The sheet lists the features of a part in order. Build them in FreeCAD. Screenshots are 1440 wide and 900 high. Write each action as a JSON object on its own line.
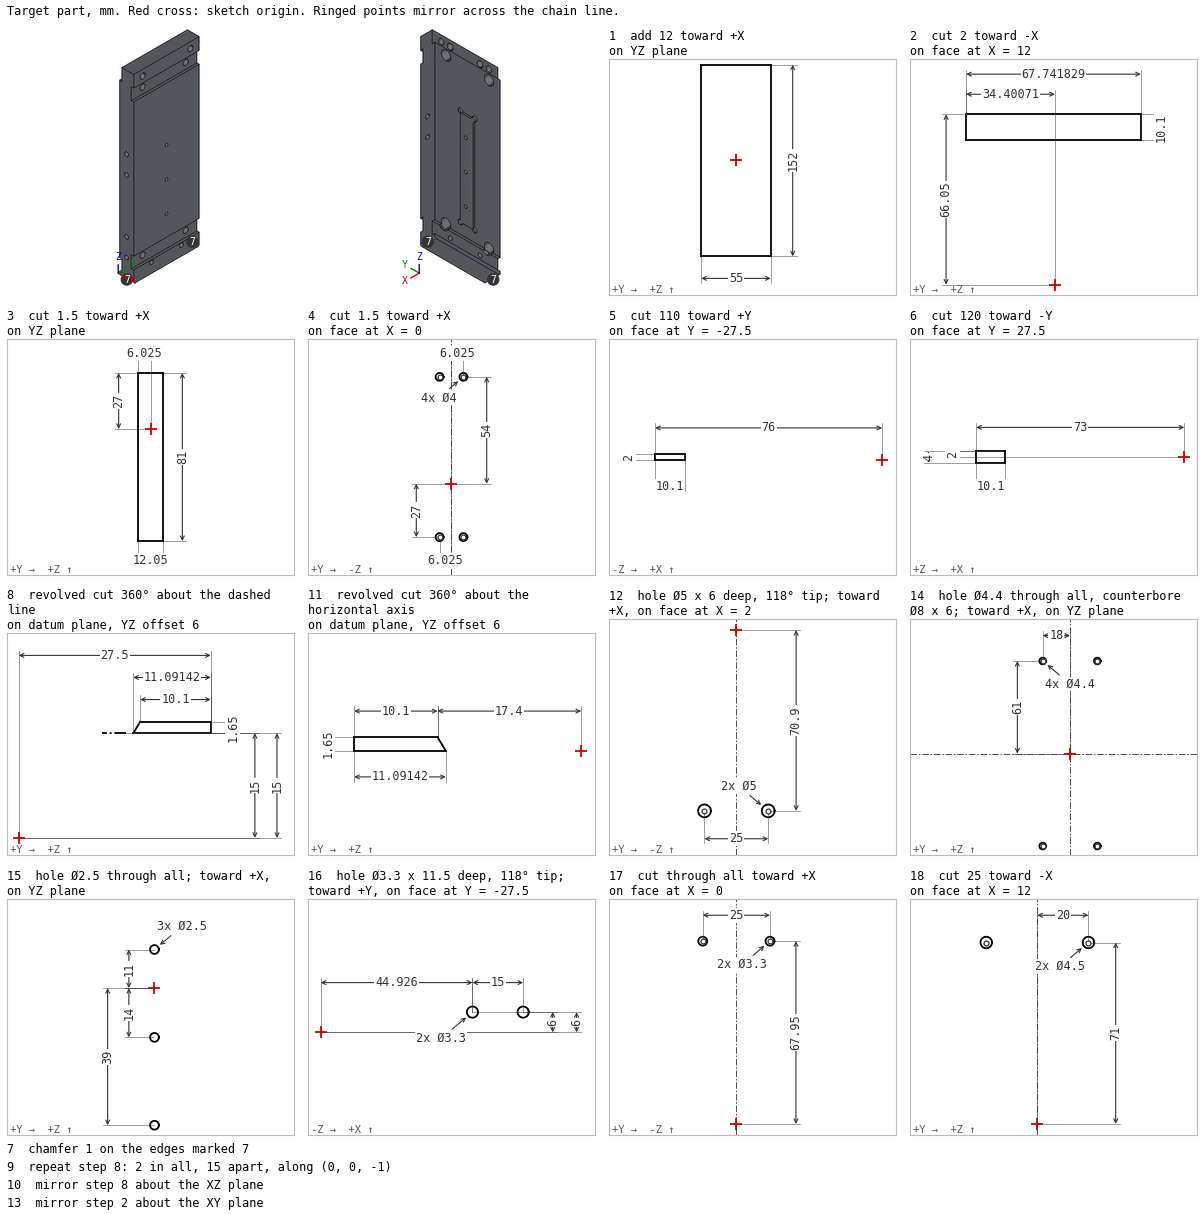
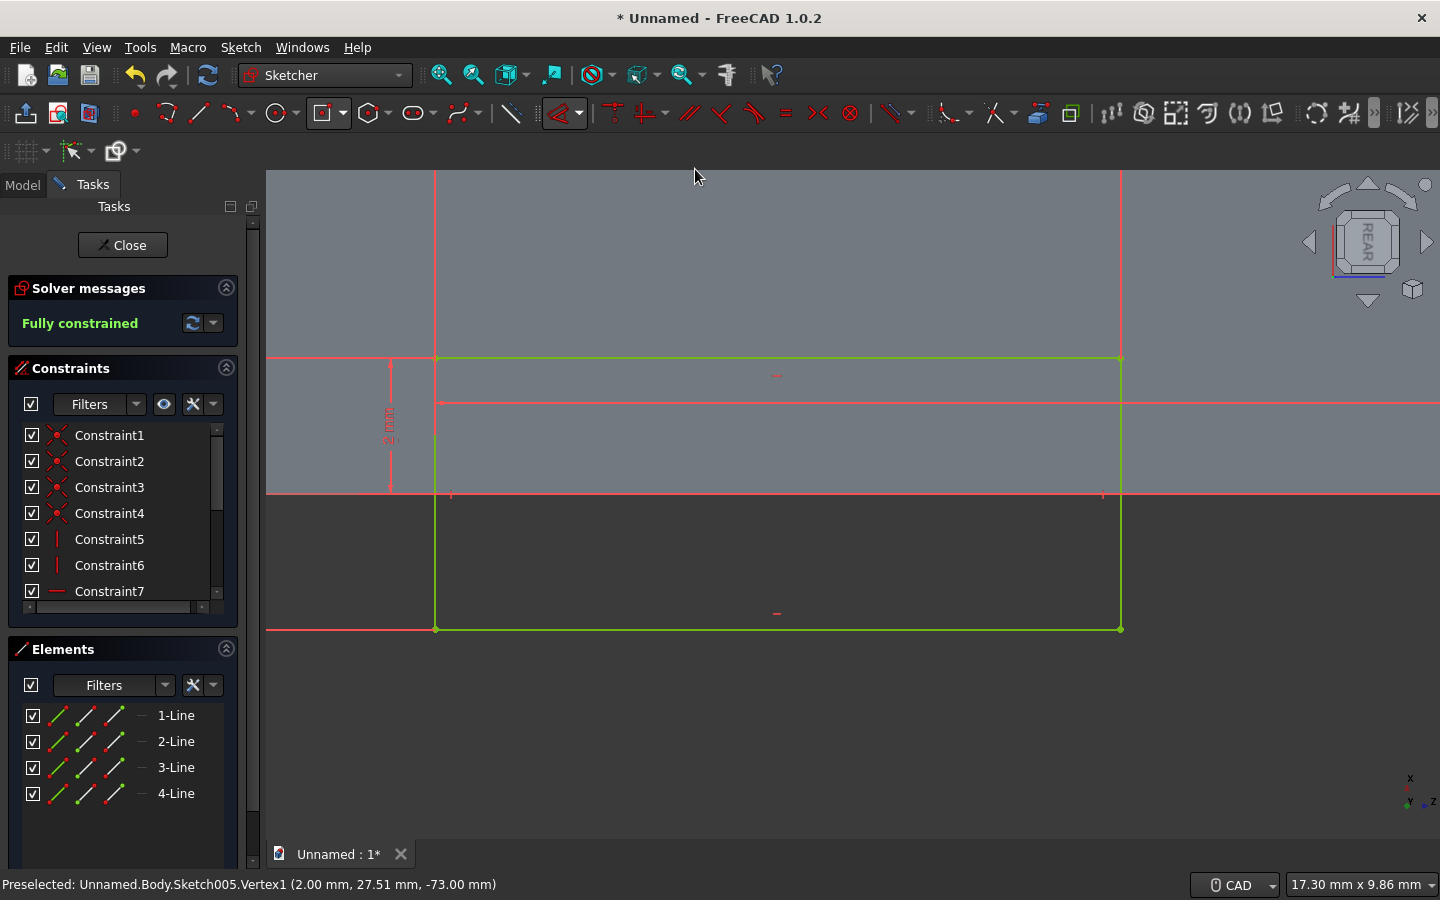
{"action": "left_click", "coordinate": [123, 245]}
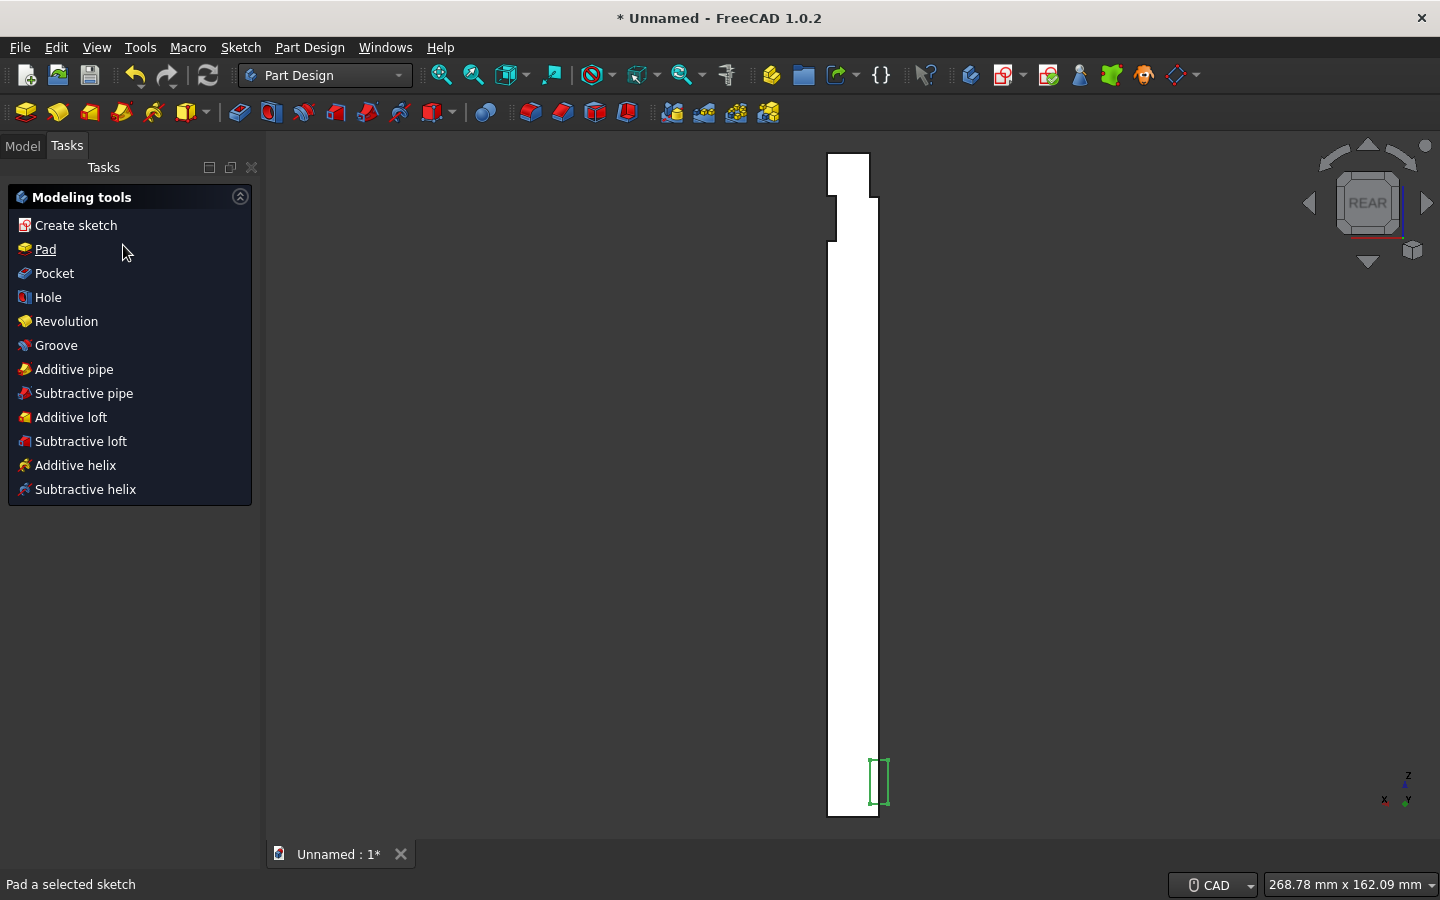
{"action": "left_click", "coordinate": [240, 112]}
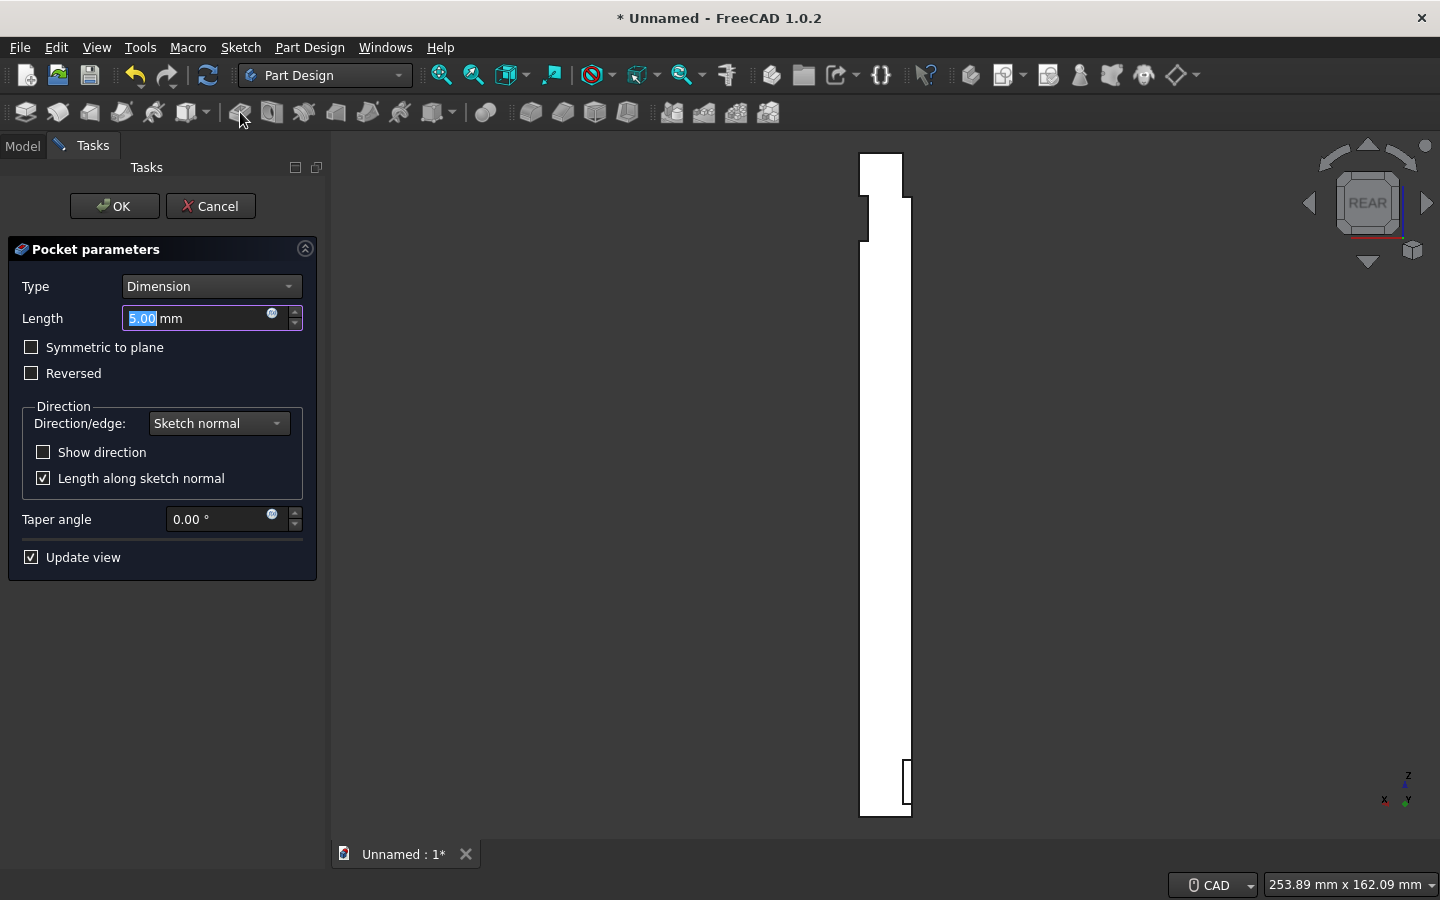
{"action": "type", "text": "120"}
{"action": "key", "text": "Tab"}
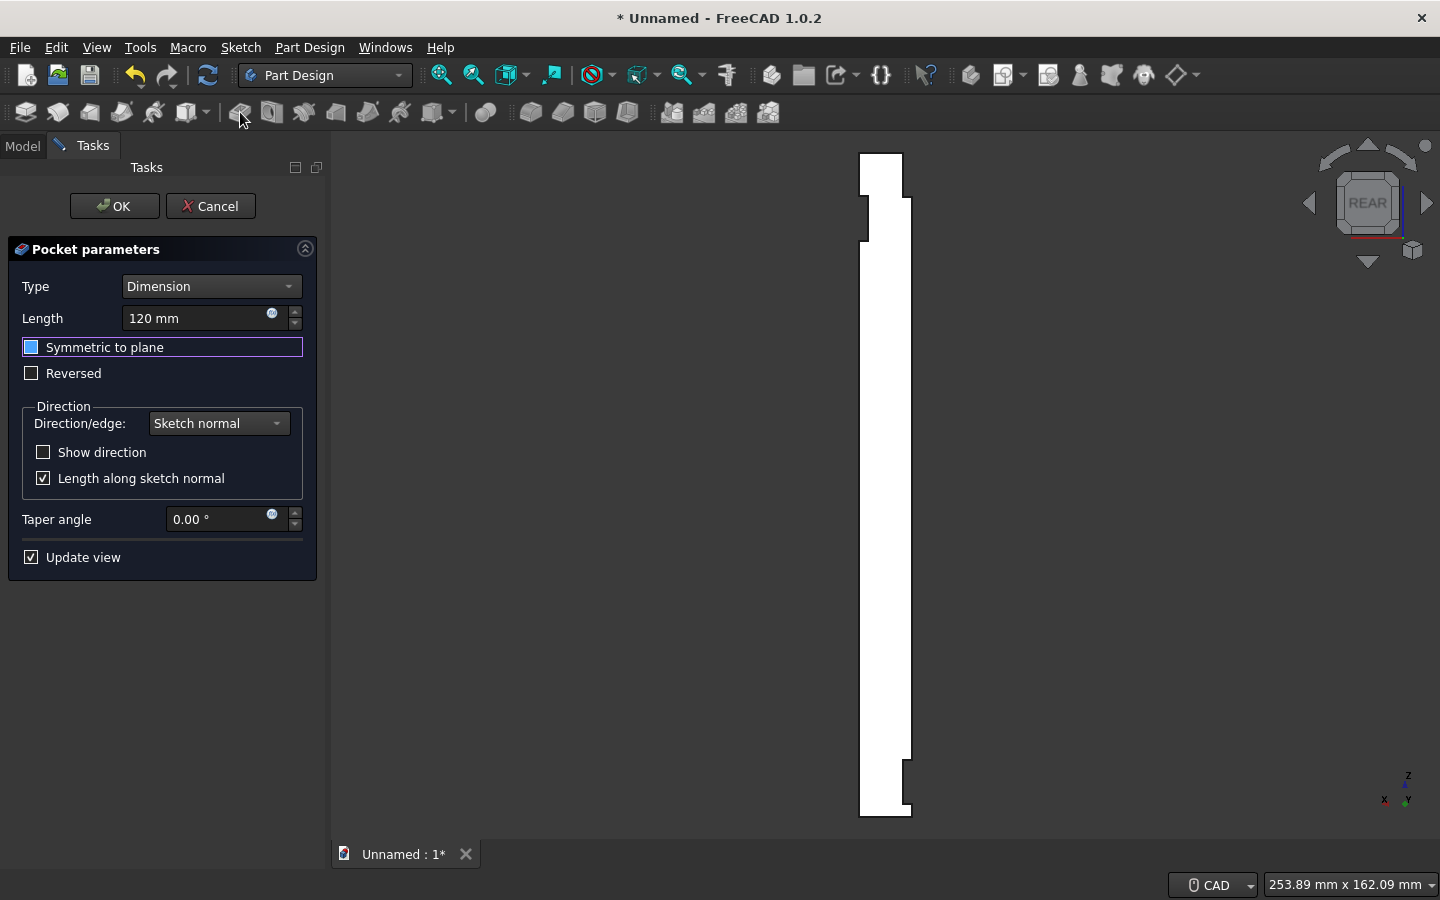
{"action": "left_click", "coordinate": [115, 206]}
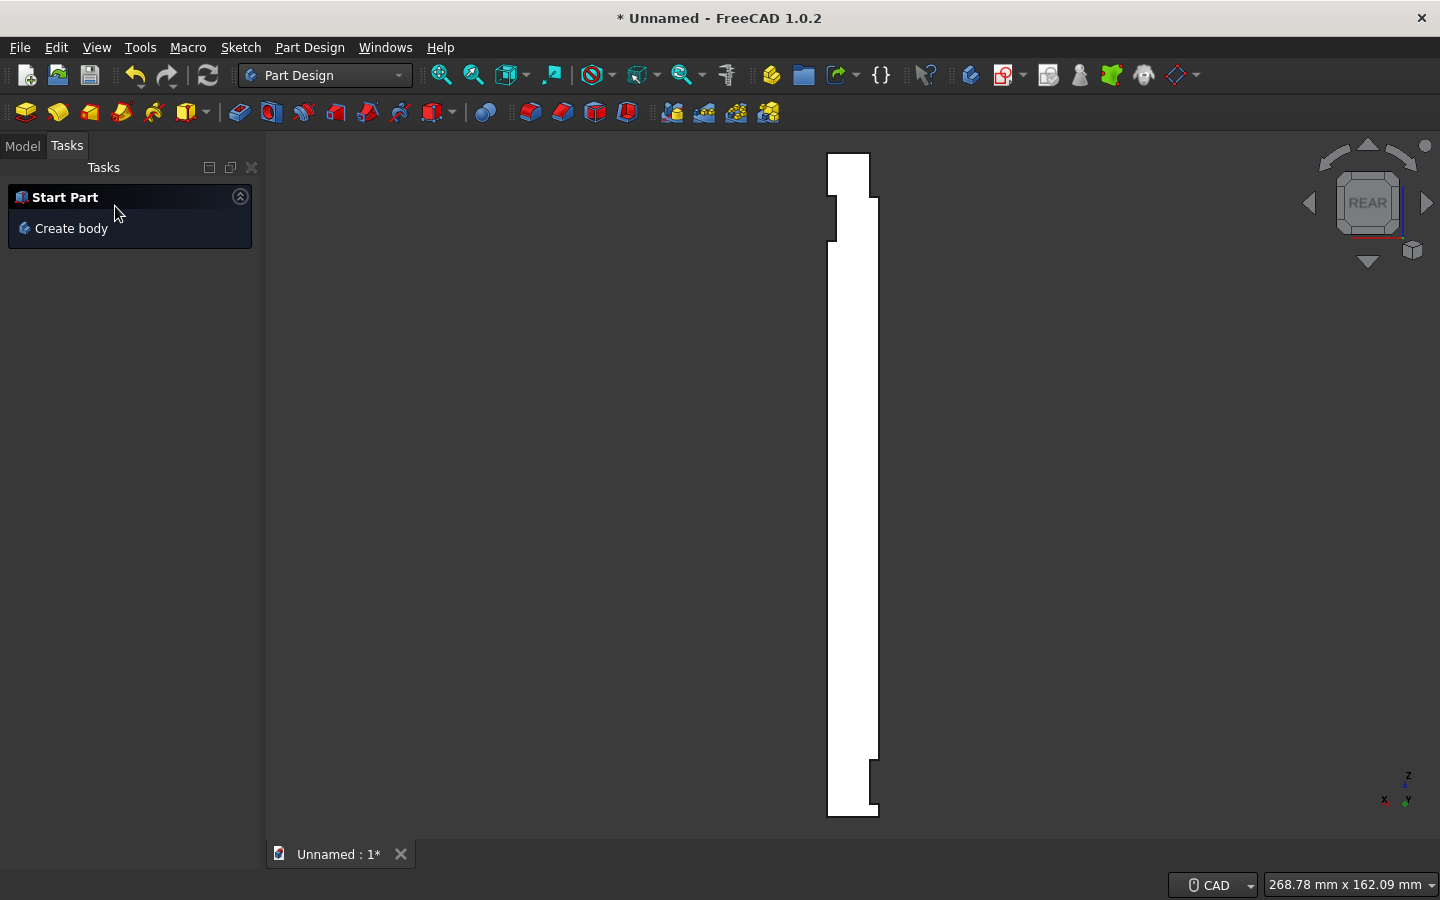
{"action": "key", "text": "0"}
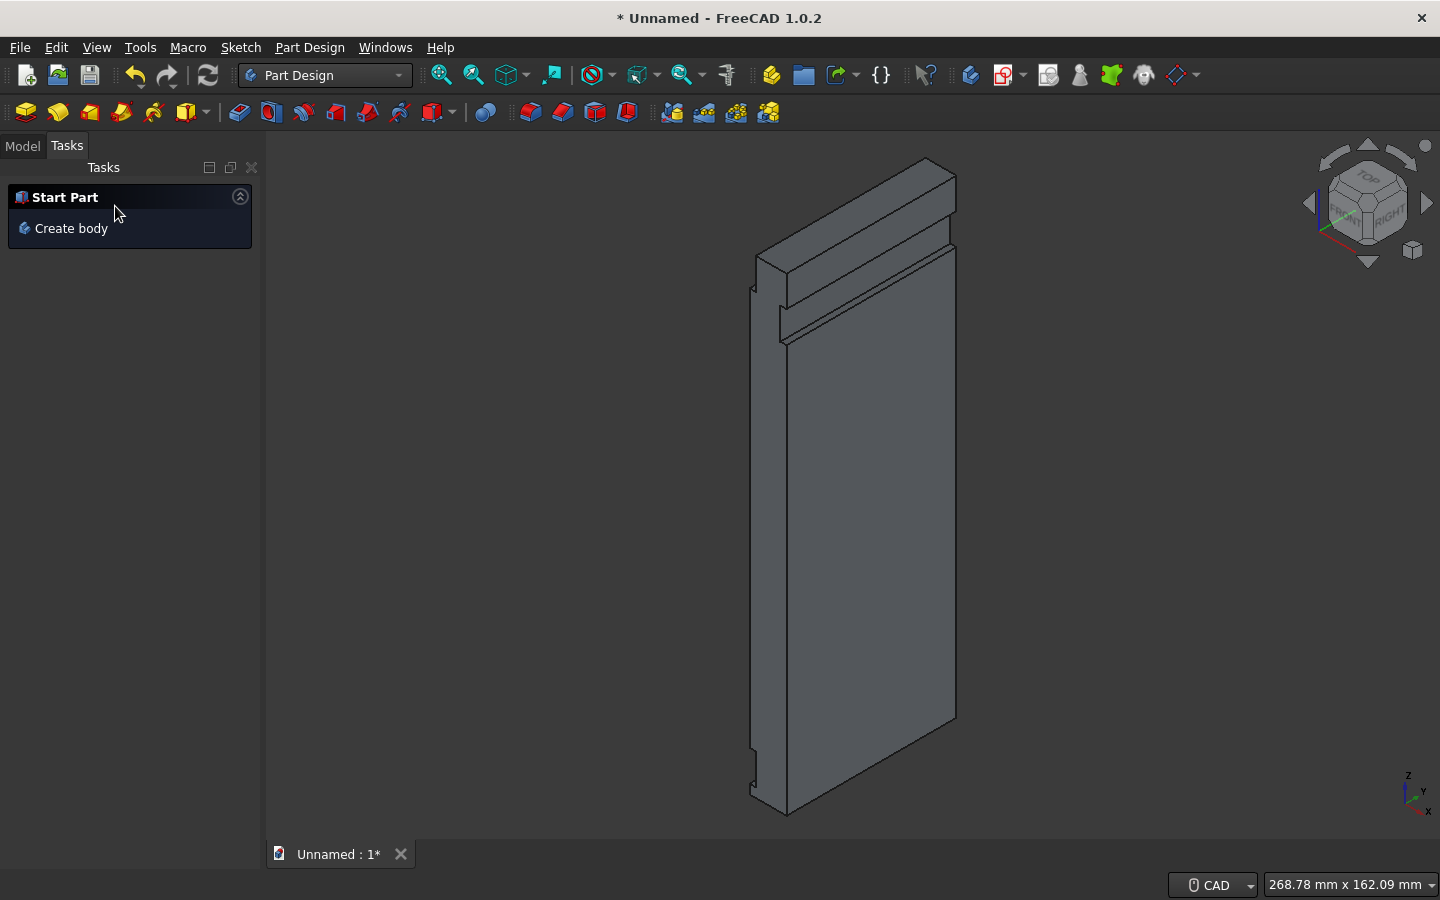
{"action": "key", "text": "2"}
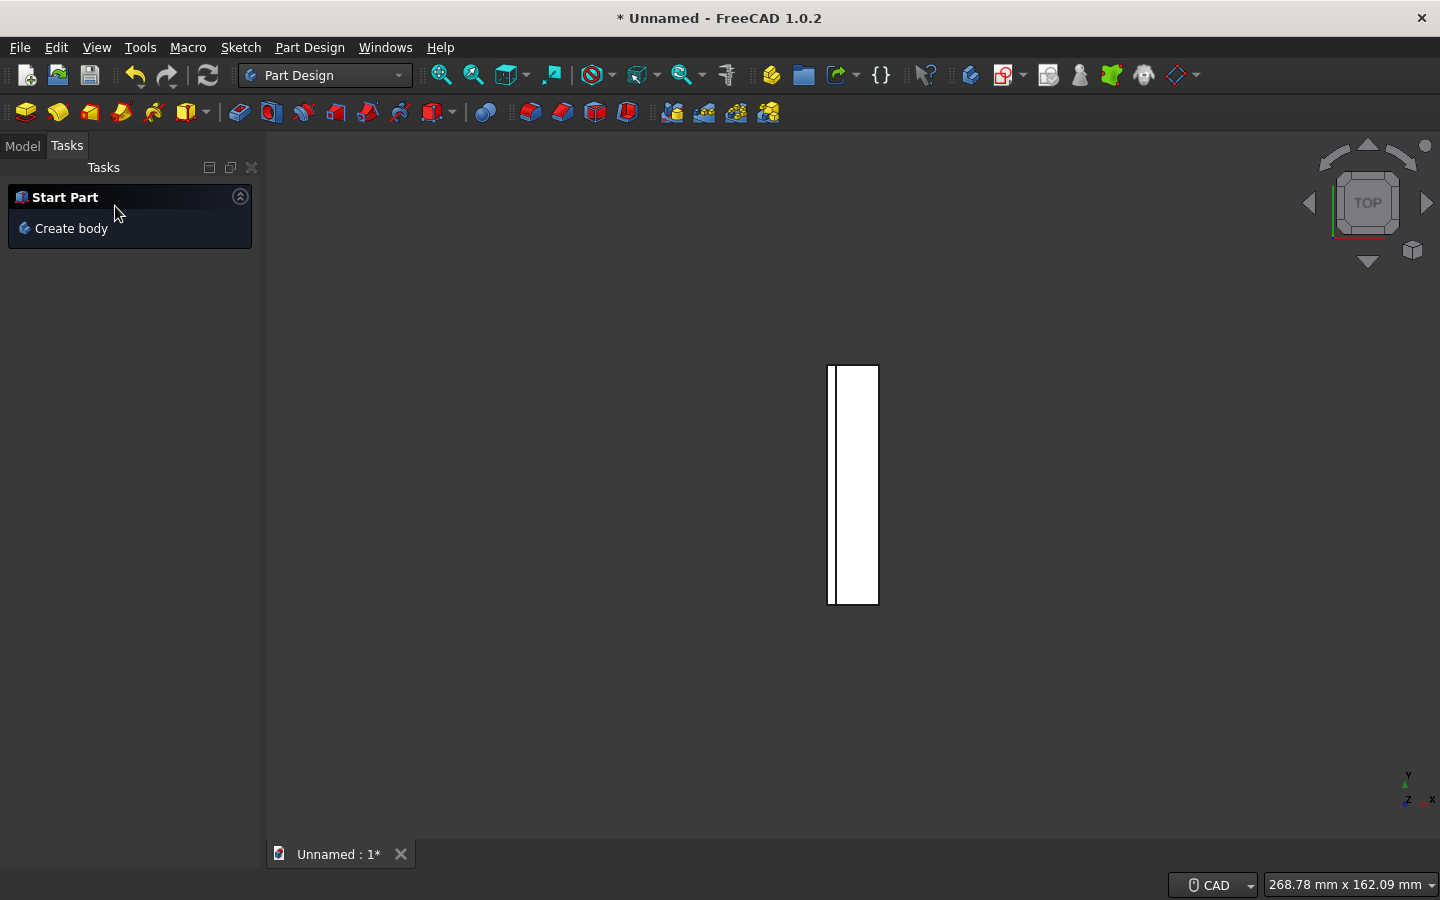
{"action": "key", "text": "v f"}